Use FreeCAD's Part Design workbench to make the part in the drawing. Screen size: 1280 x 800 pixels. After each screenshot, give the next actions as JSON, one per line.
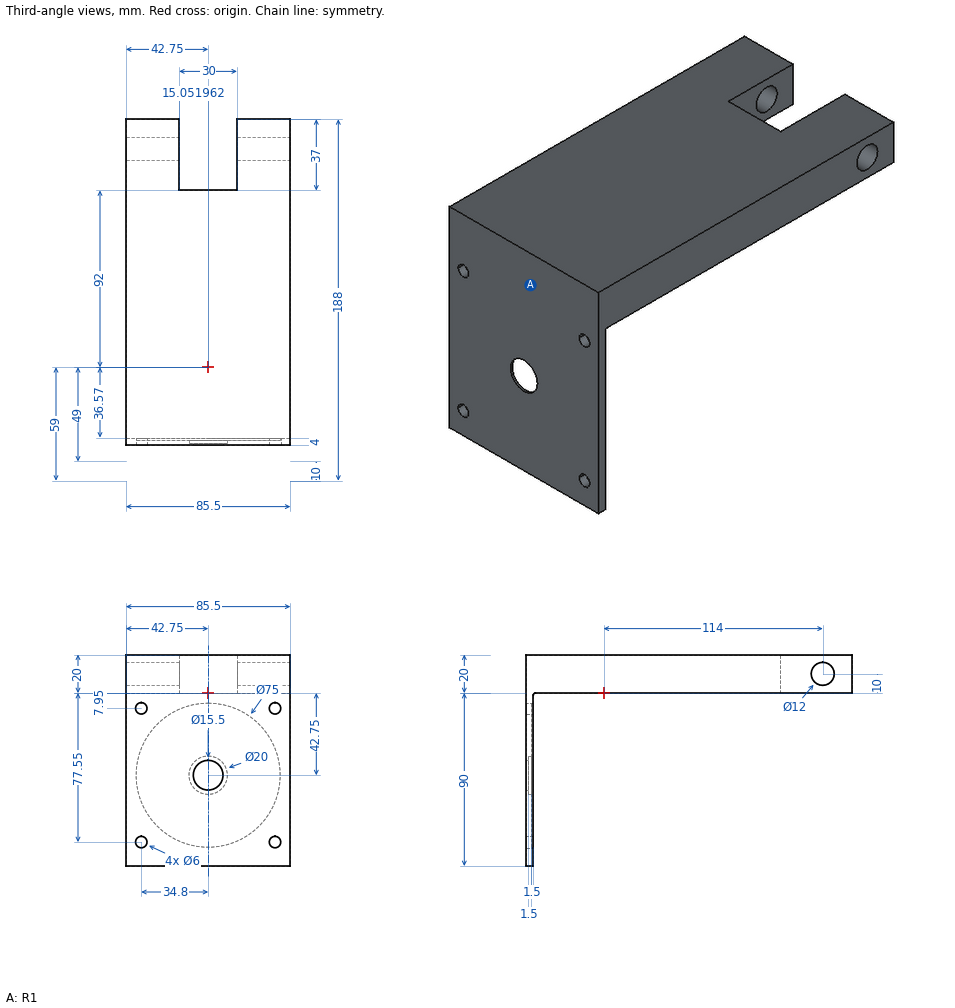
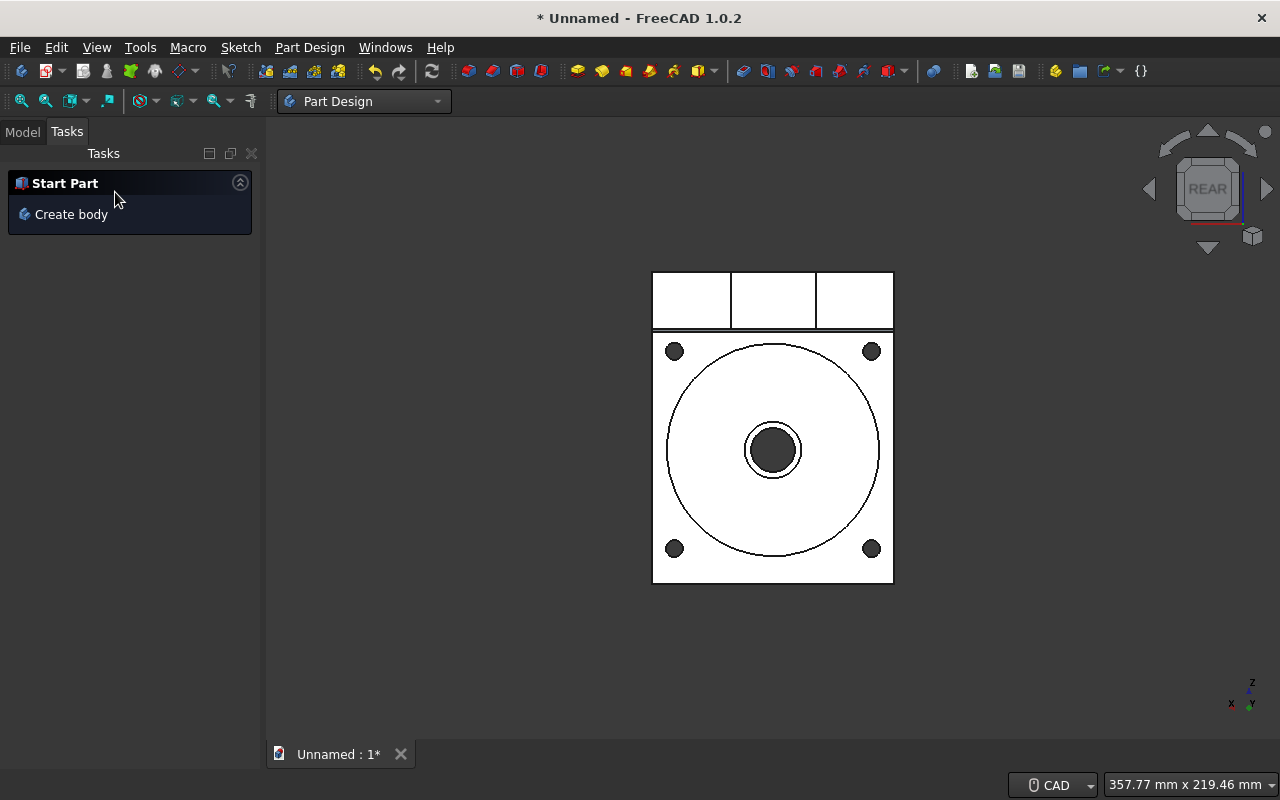
{"action": "key", "text": "0"}